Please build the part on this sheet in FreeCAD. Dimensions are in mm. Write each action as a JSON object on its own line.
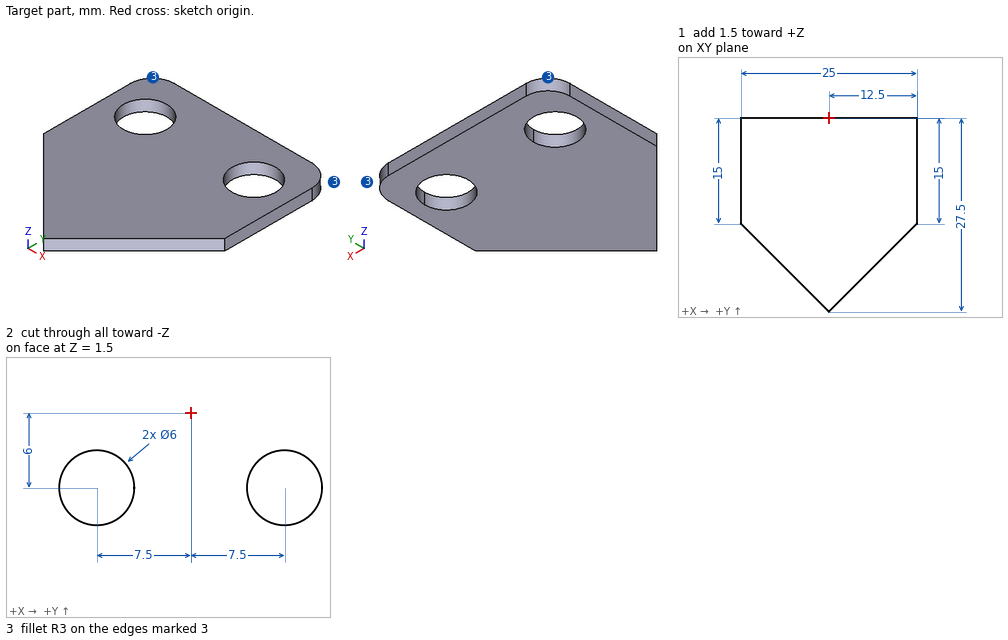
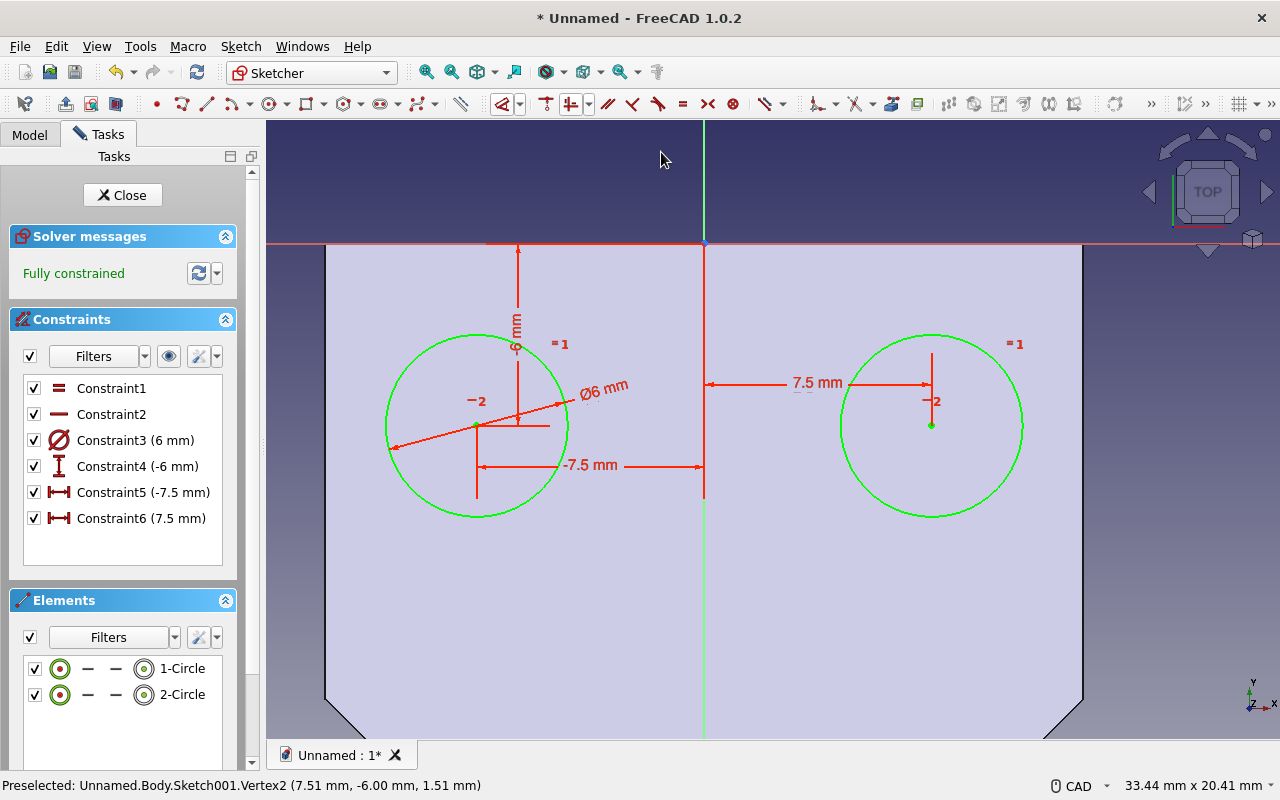
{"action": "left_click", "coordinate": [123, 195]}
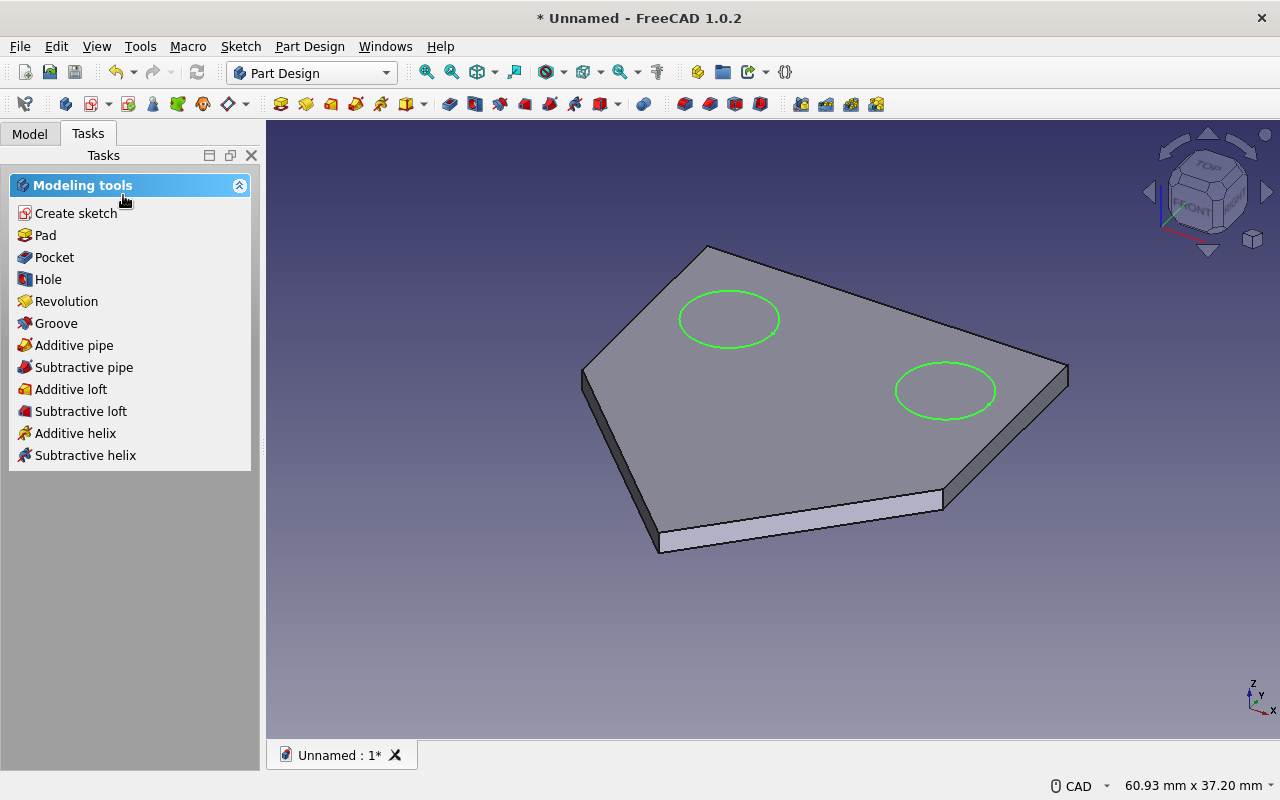
{"action": "left_click", "coordinate": [450, 104]}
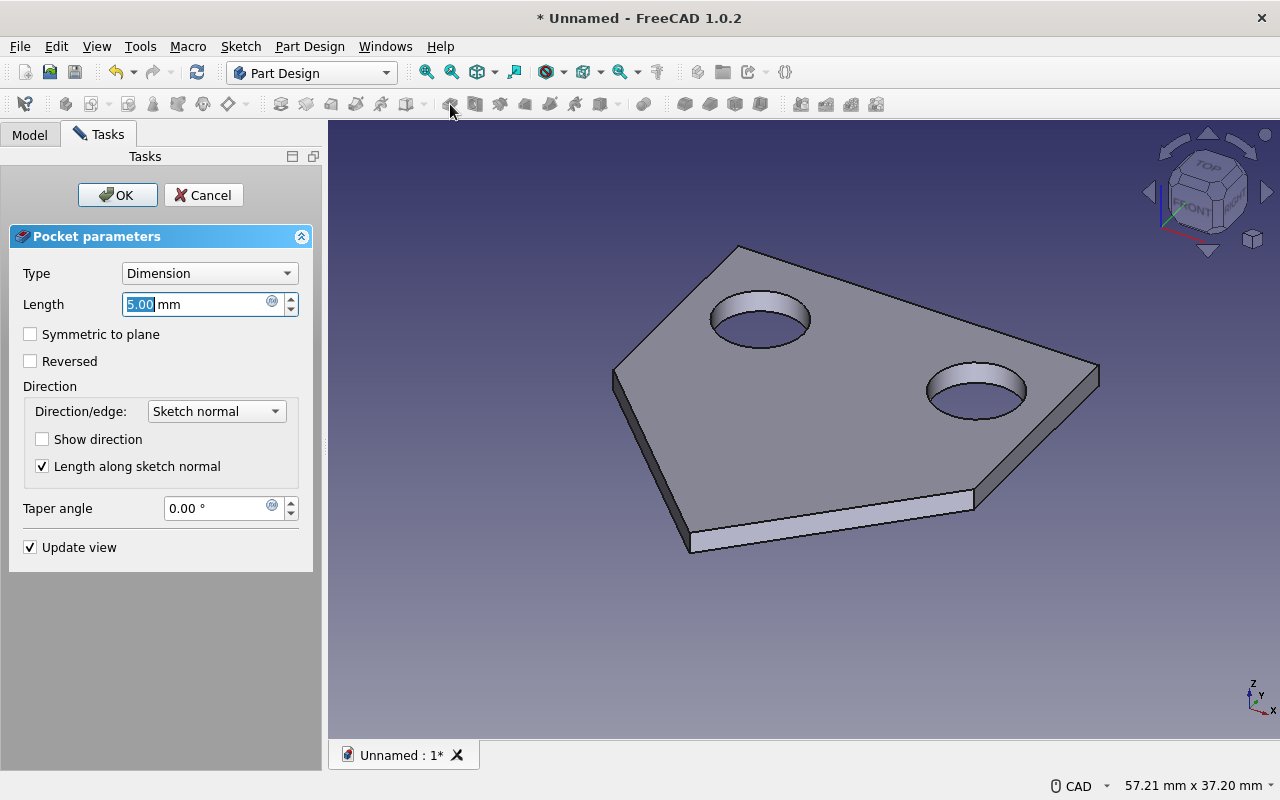
{"action": "left_click", "coordinate": [210, 274]}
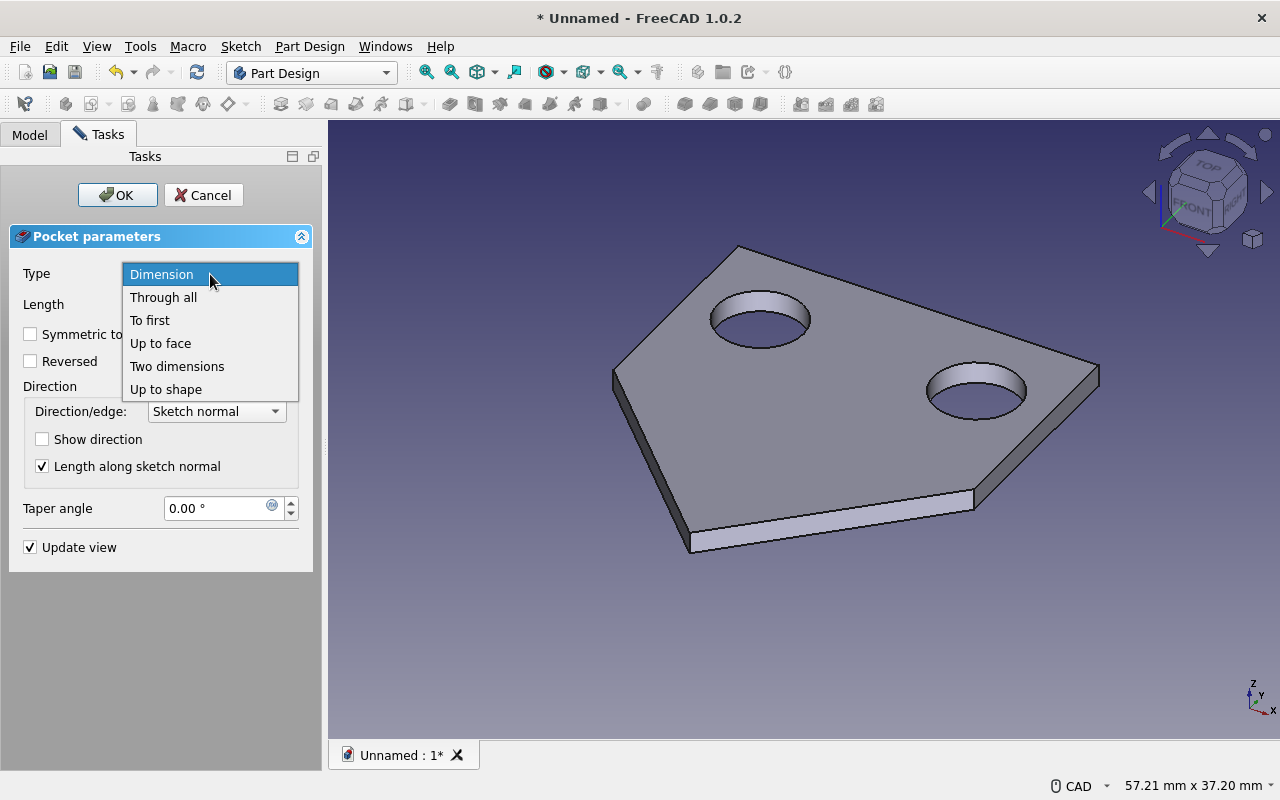
{"action": "left_click", "coordinate": [208, 298]}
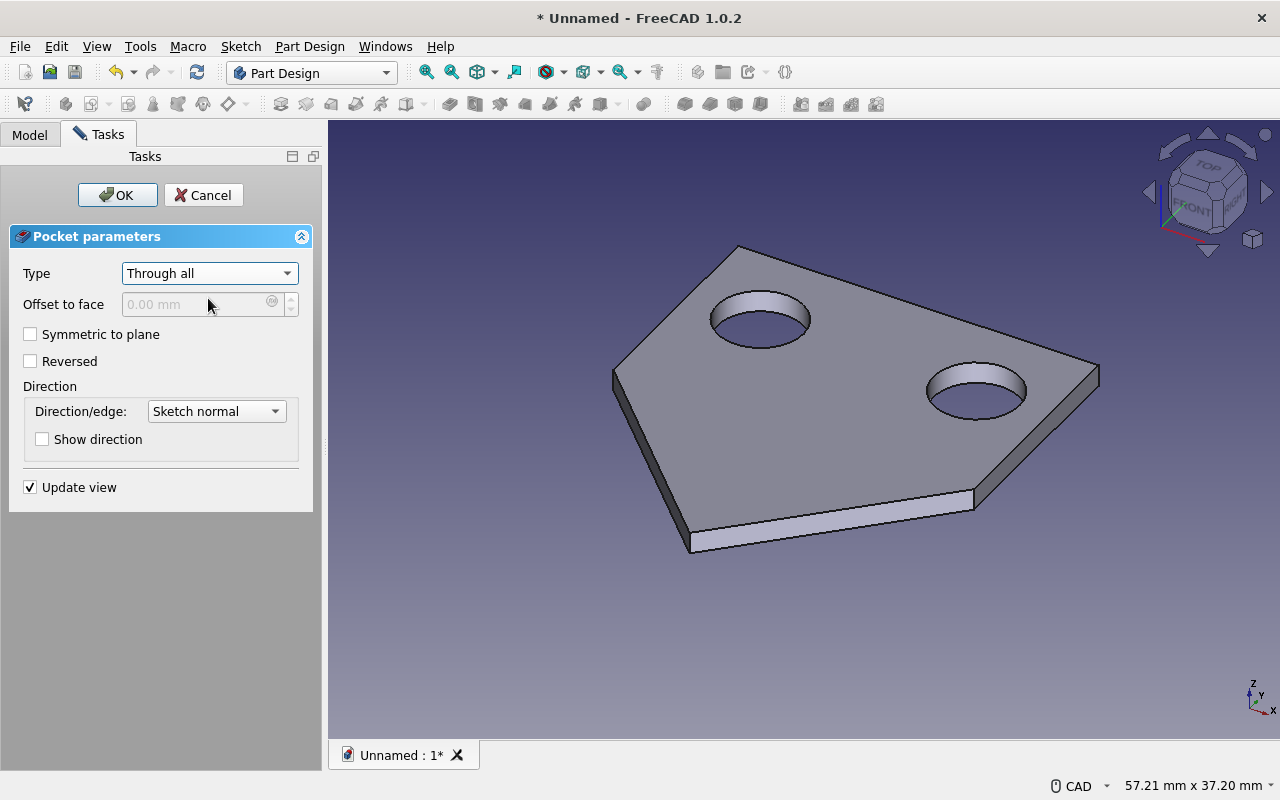
{"action": "left_click", "coordinate": [118, 195]}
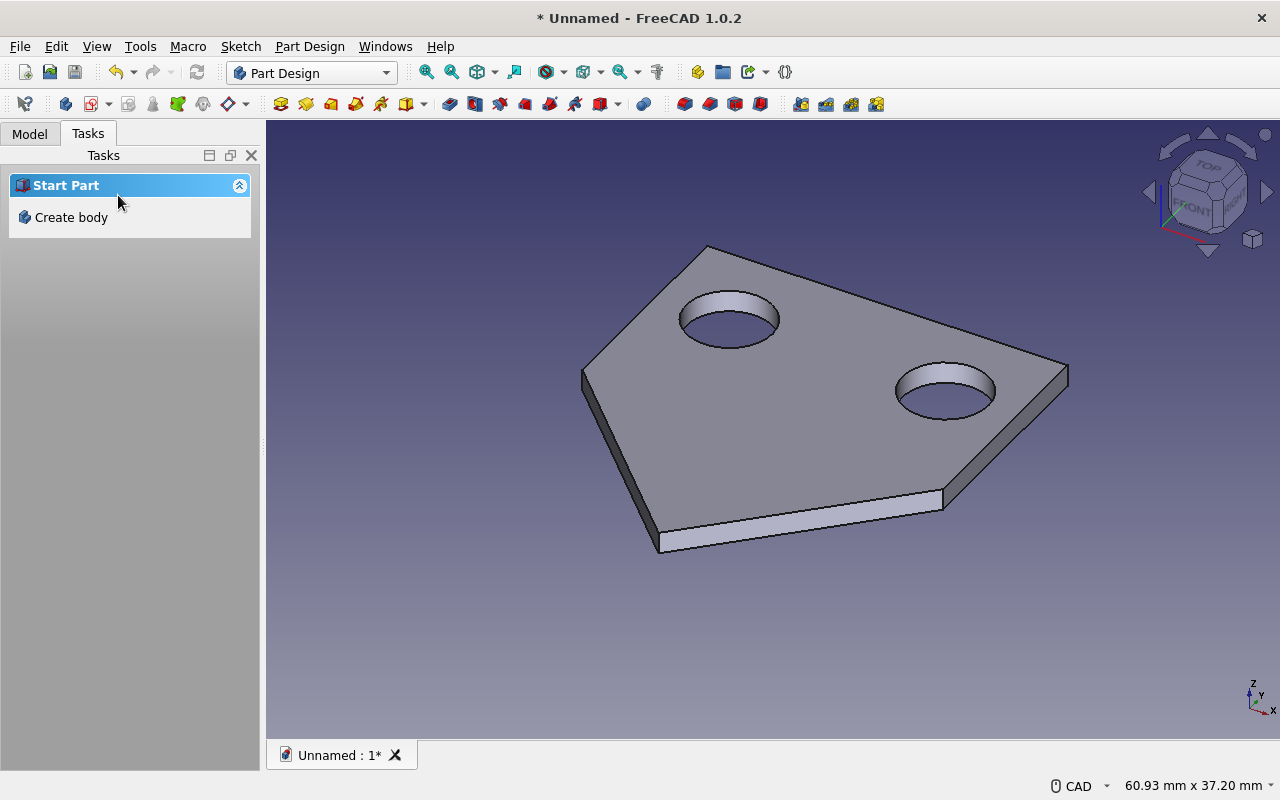
{"action": "key", "text": "0"}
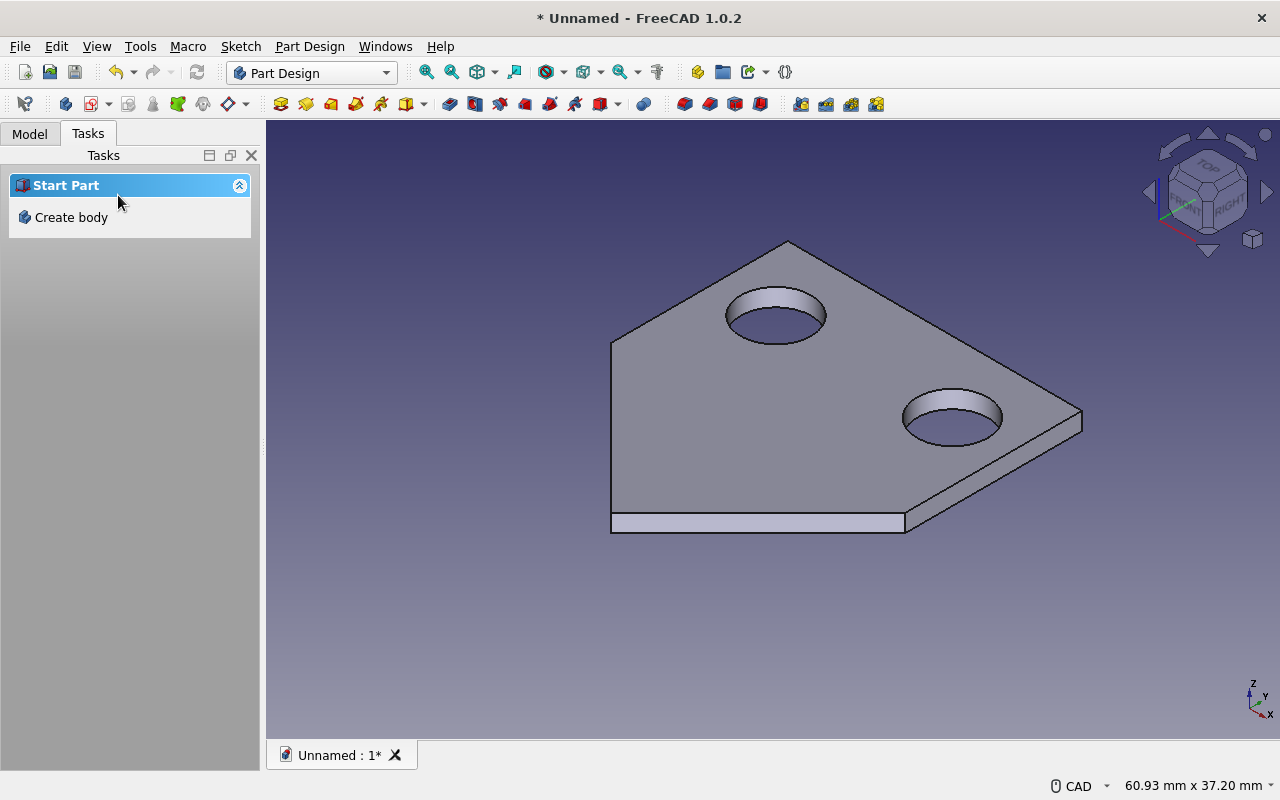
{"action": "key", "text": "2"}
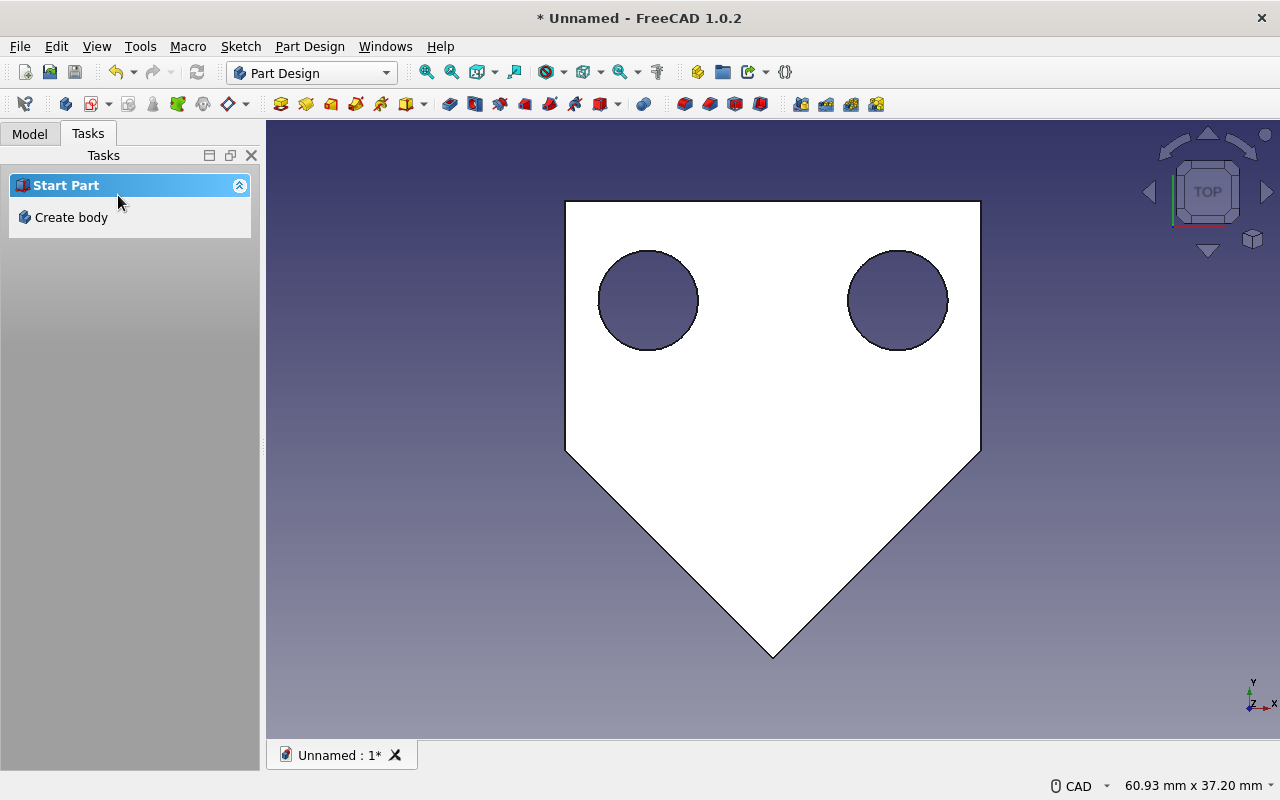
{"action": "key", "text": "1"}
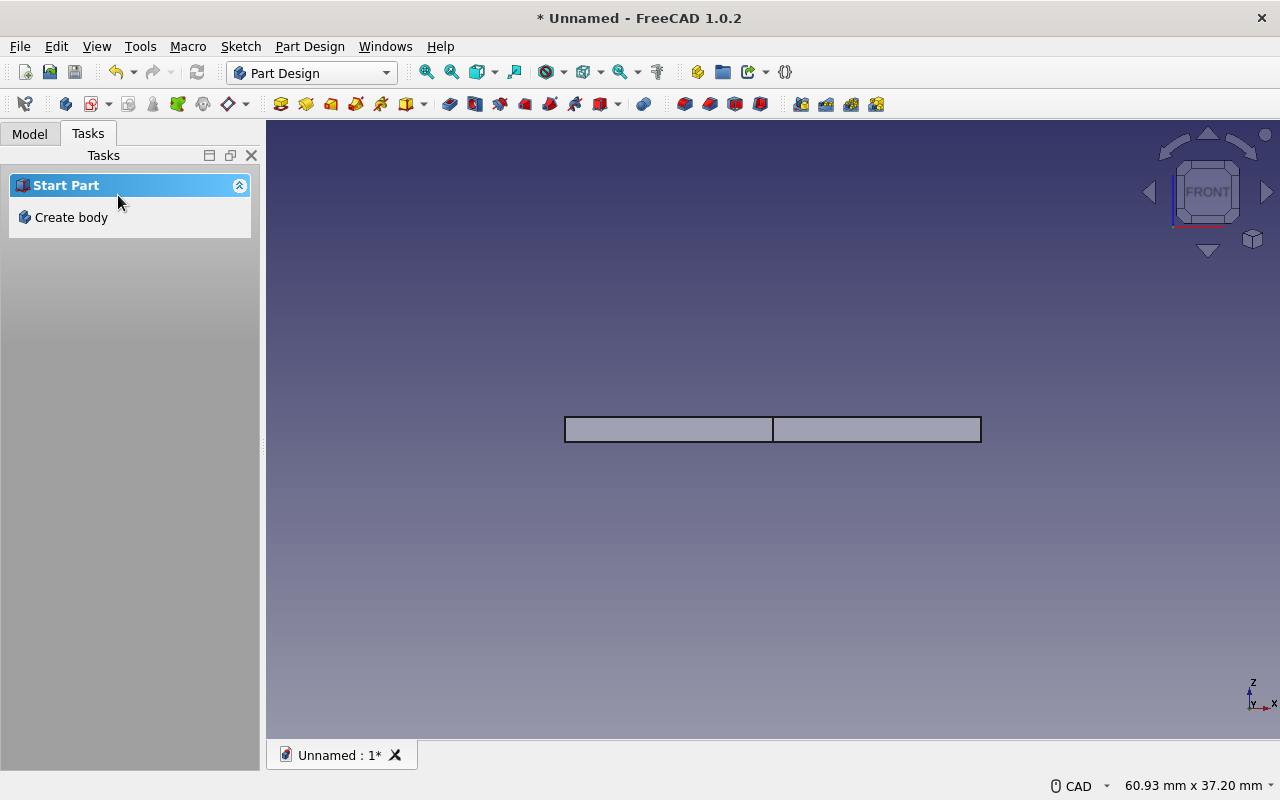
{"action": "left_click", "coordinate": [427, 72]}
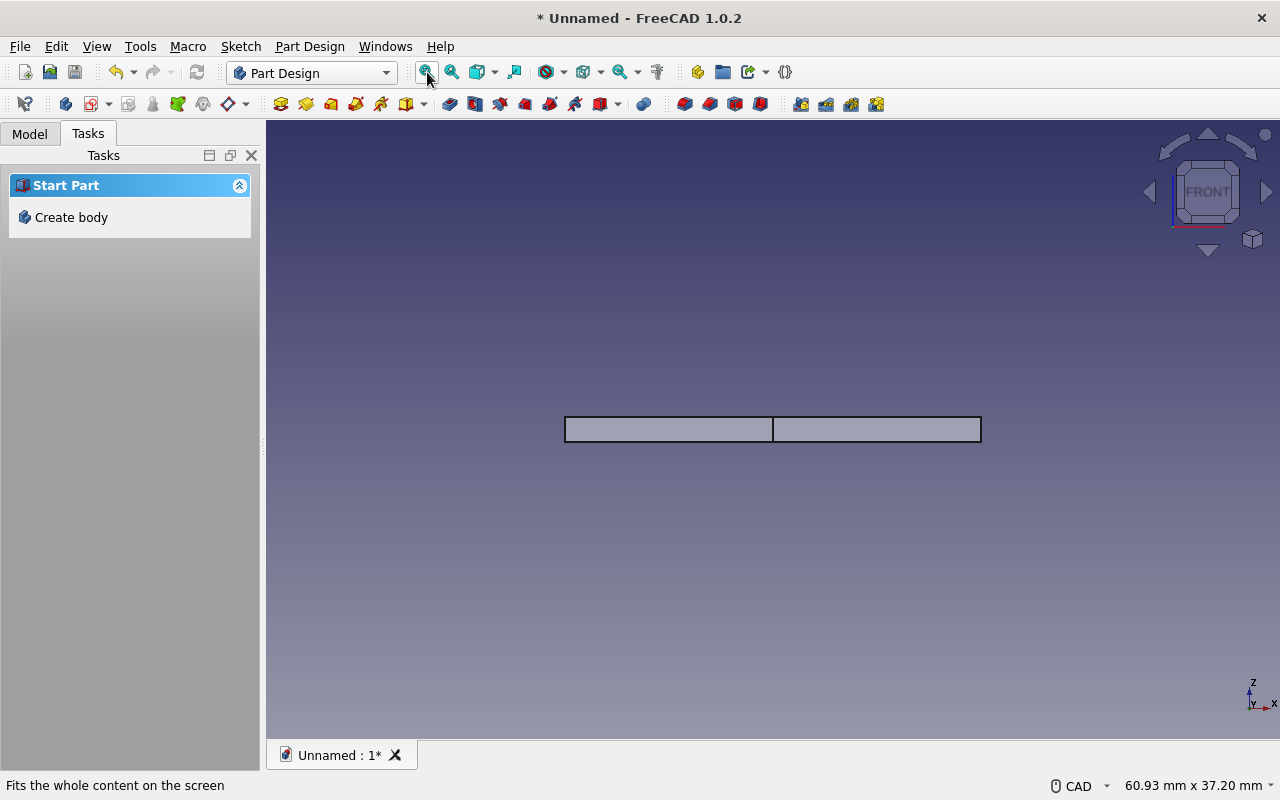
{"action": "key", "text": "3"}